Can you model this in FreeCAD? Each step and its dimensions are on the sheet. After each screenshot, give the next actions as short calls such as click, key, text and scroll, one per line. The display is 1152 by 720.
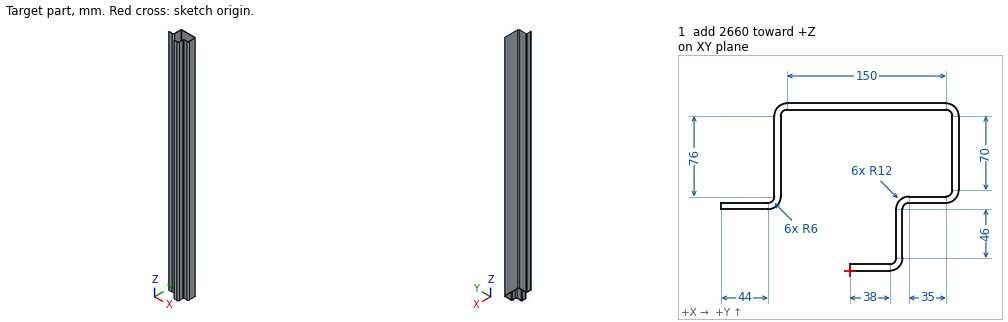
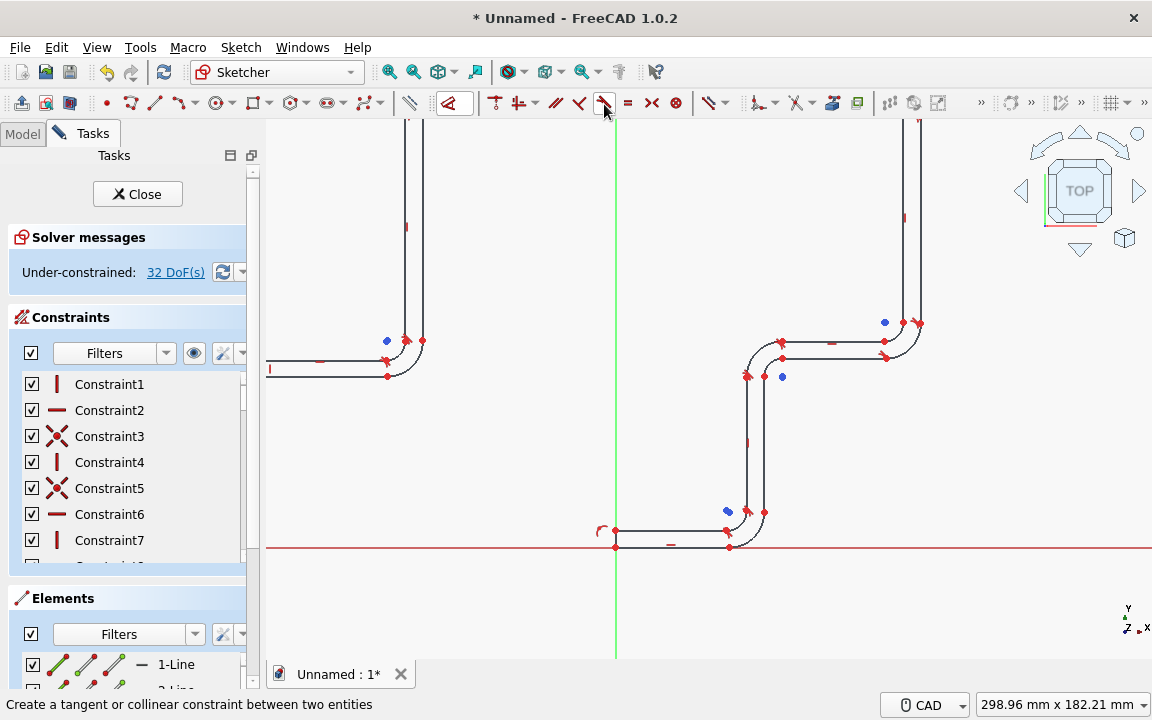
click(813, 359)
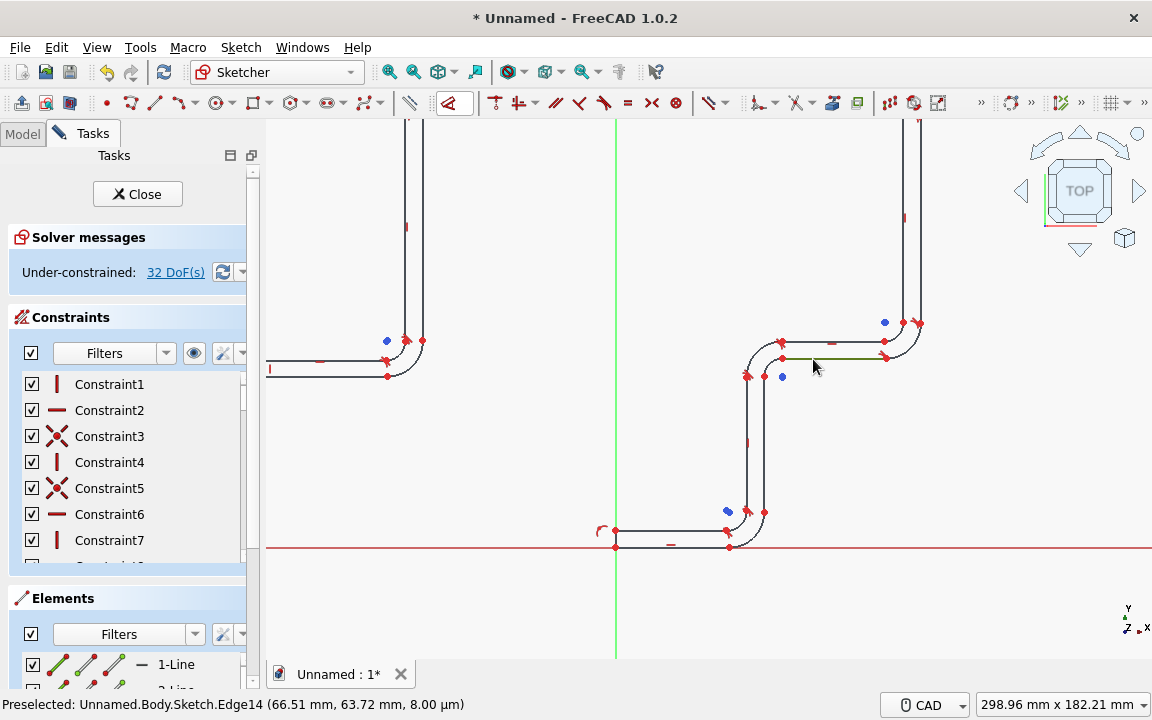
click(902, 355)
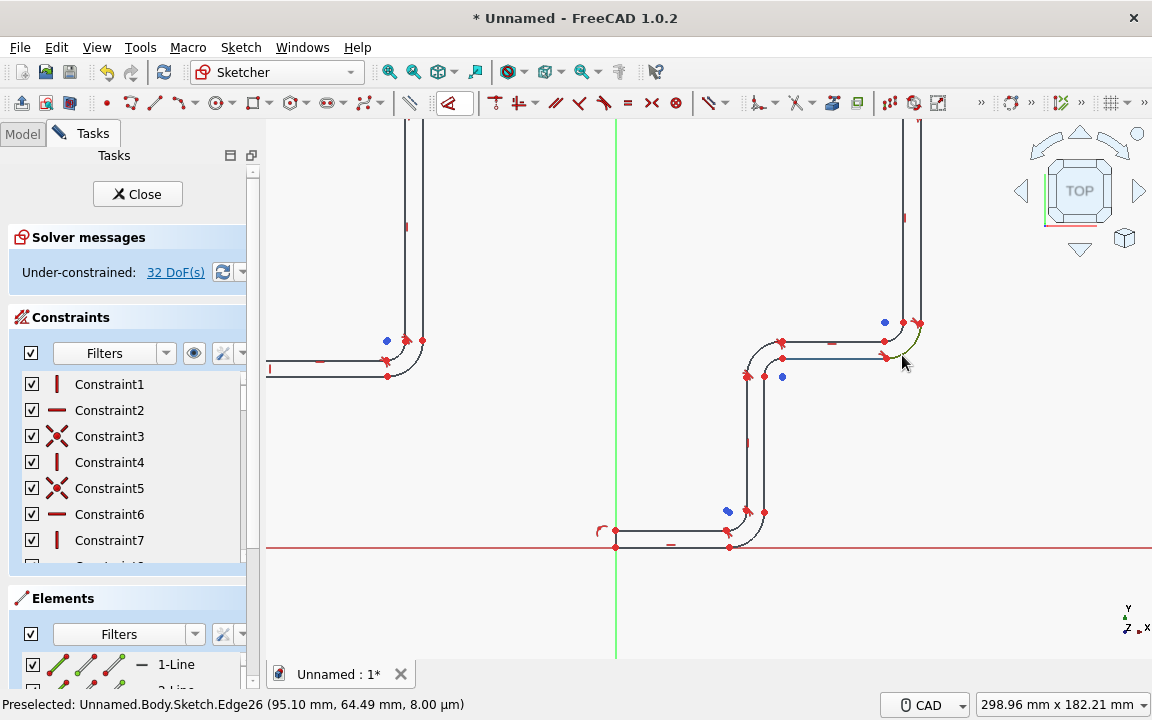
key(t)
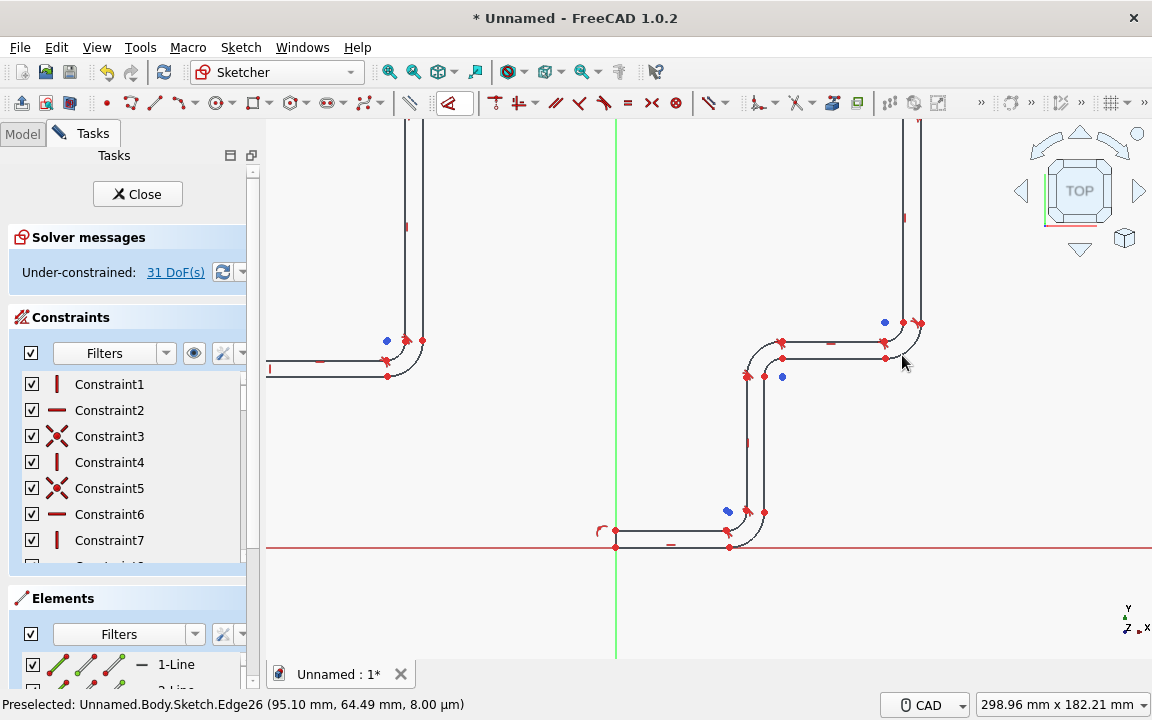
click(921, 261)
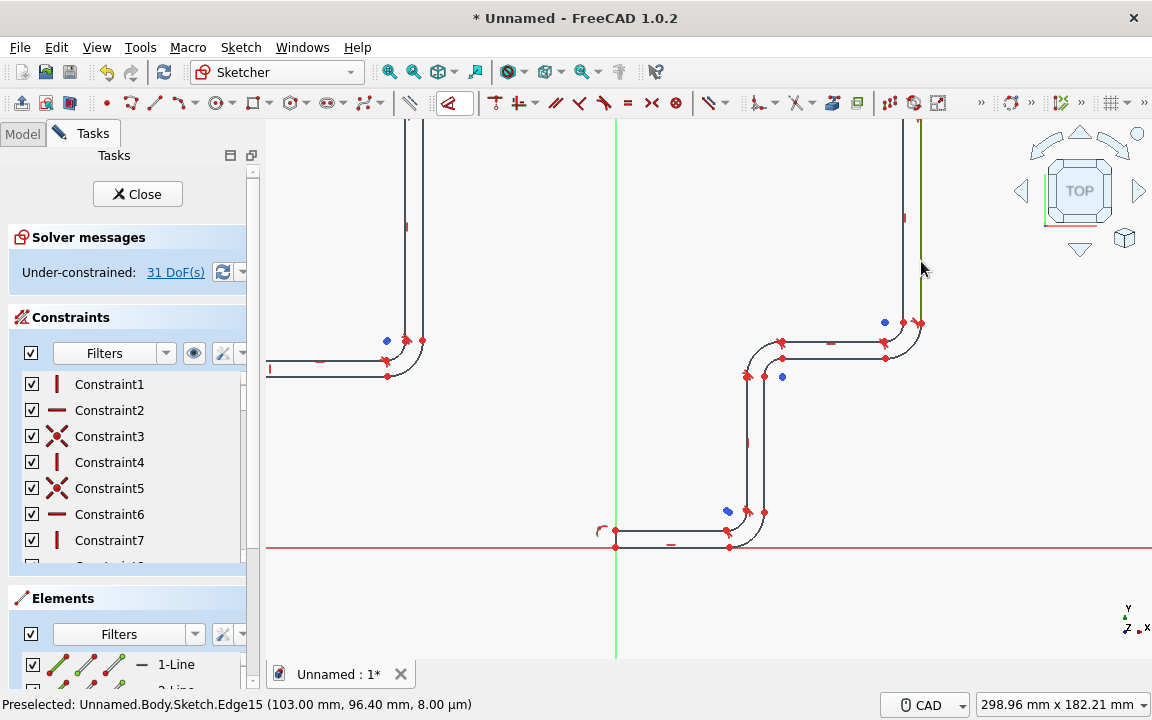
click(901, 355)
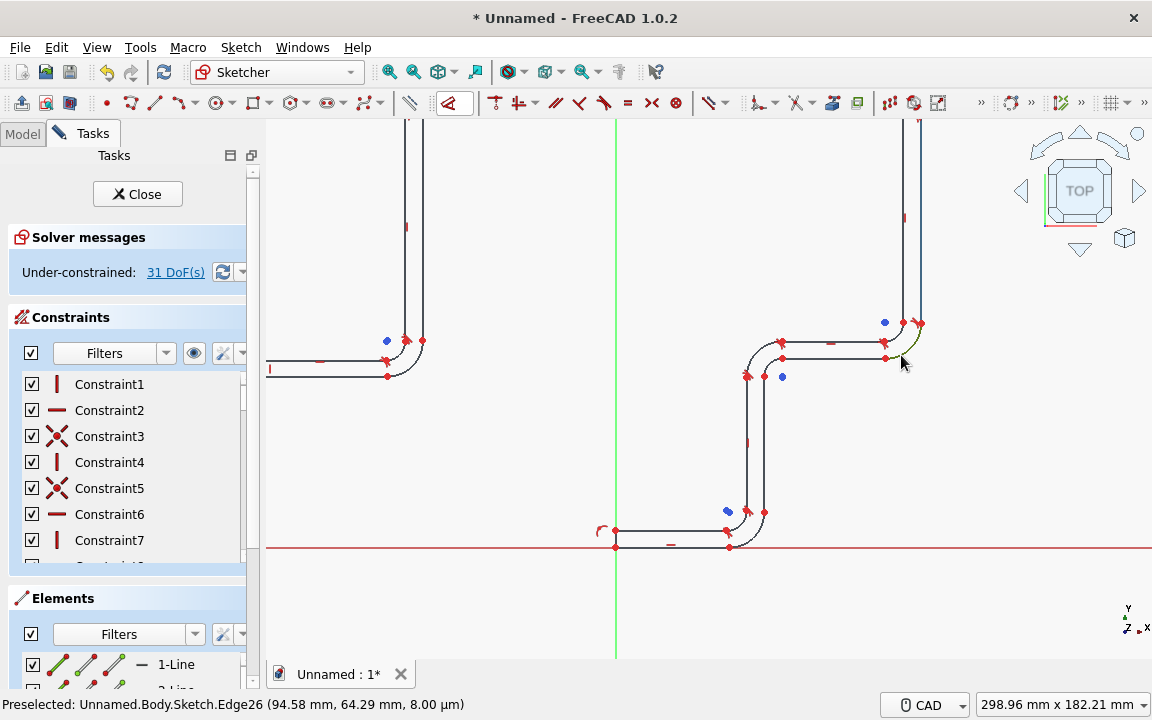
key(t)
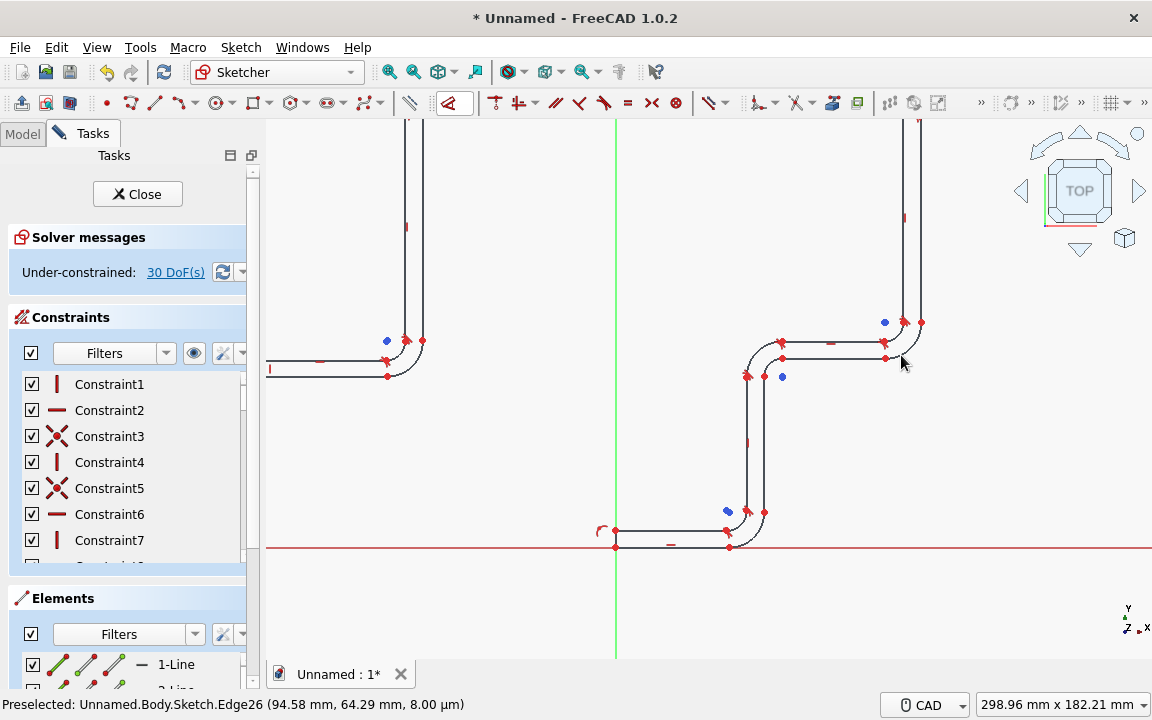
click(921, 261)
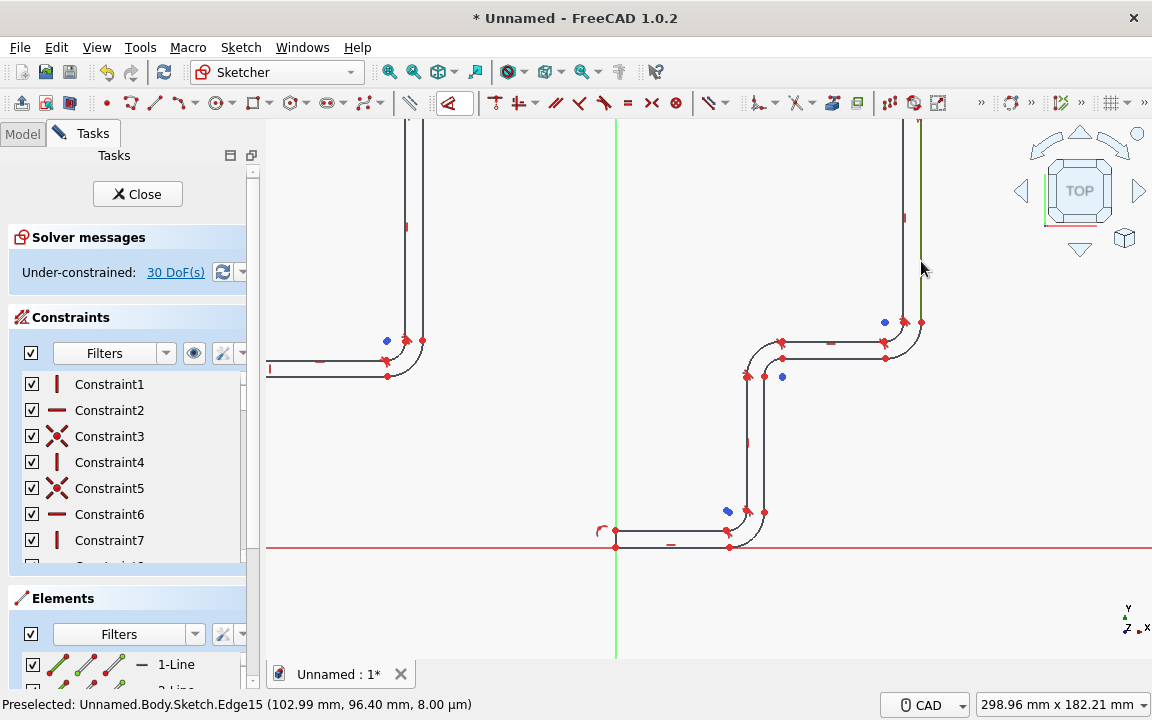
scroll(745, 542, down, 2)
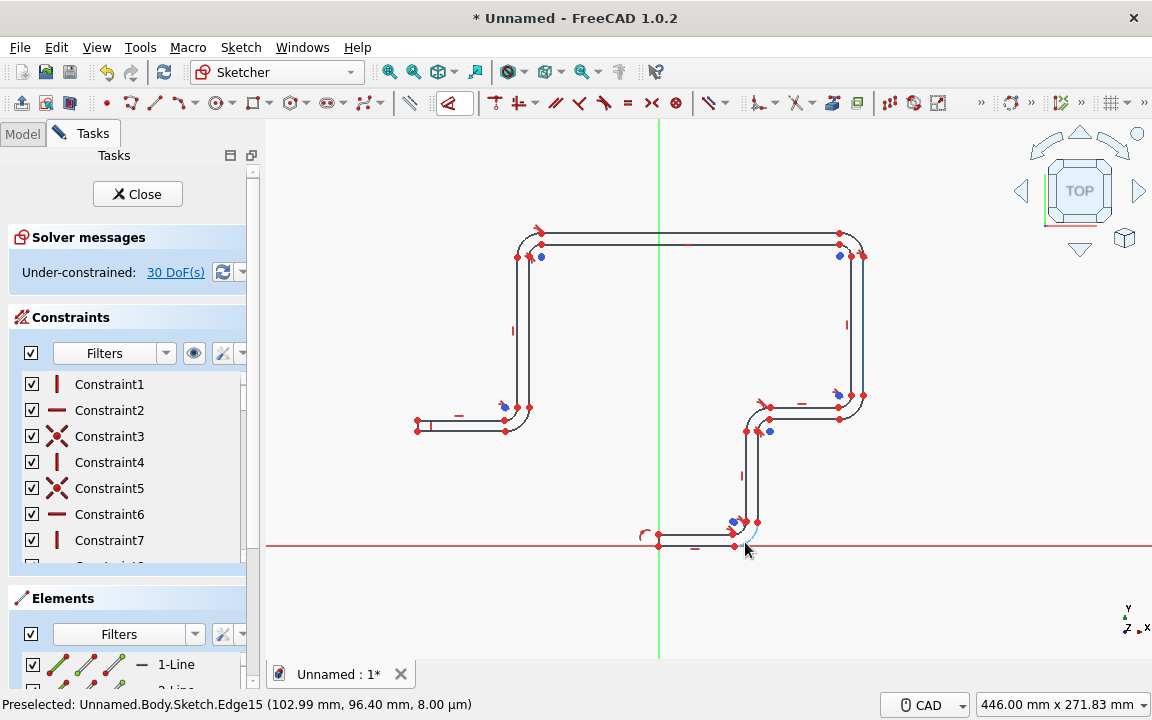
scroll(861, 246, up, 2)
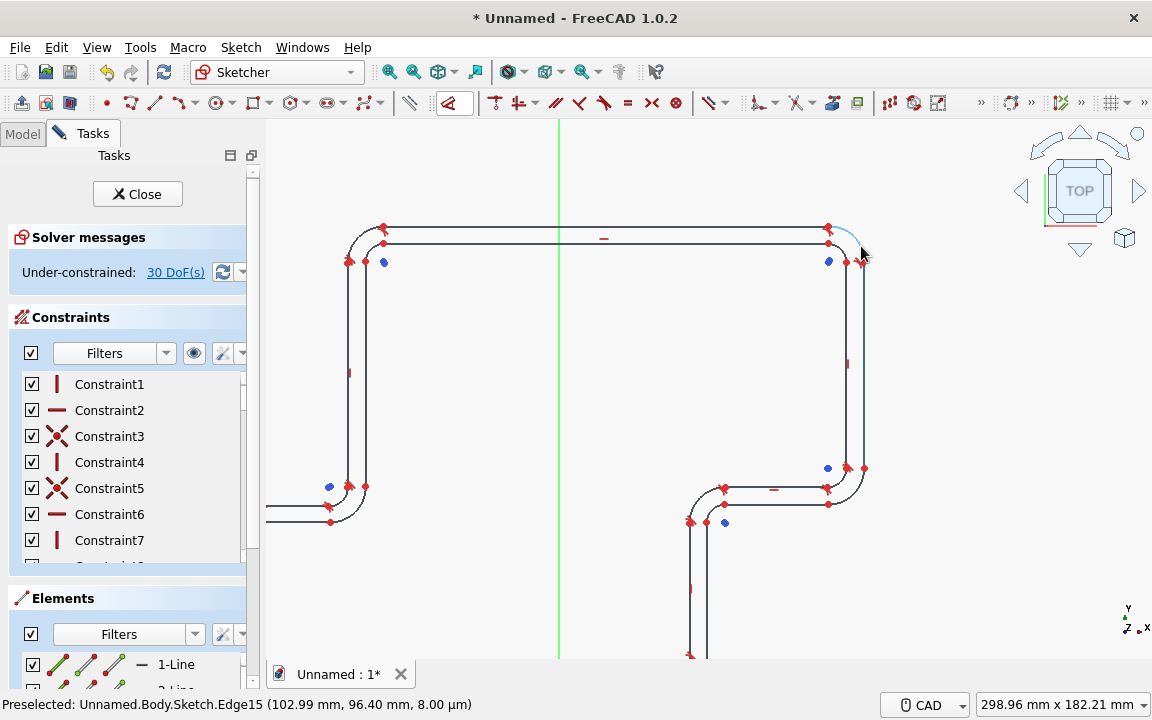
click(861, 246)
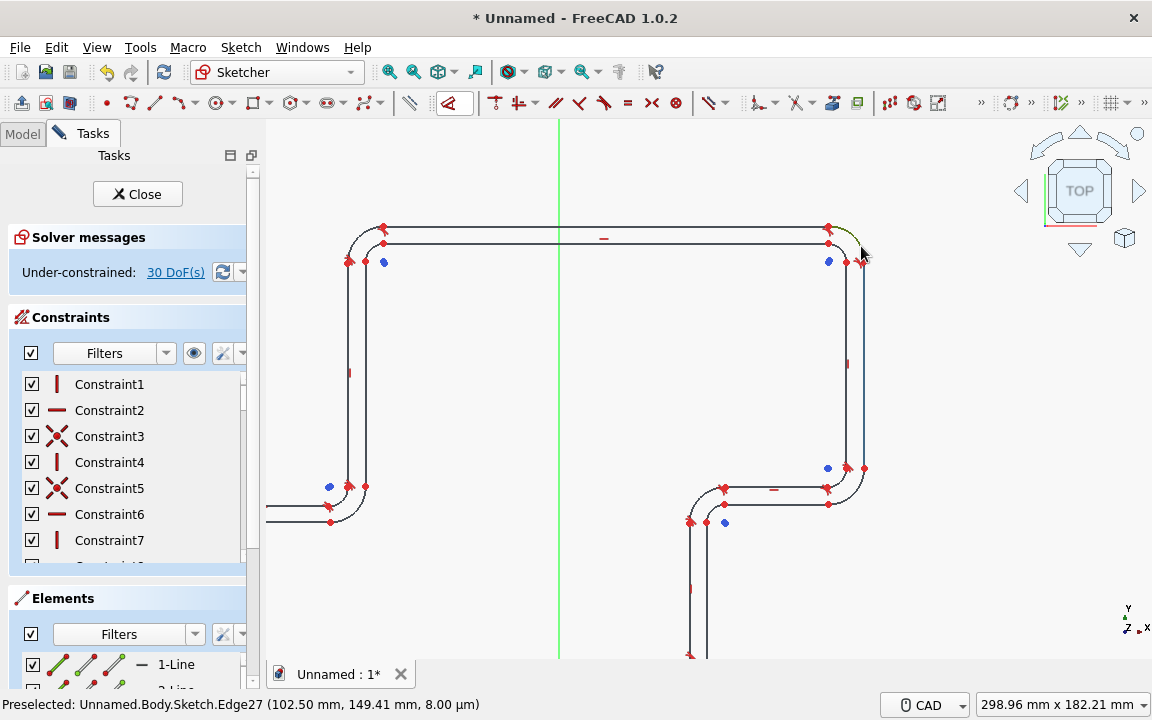
key(t)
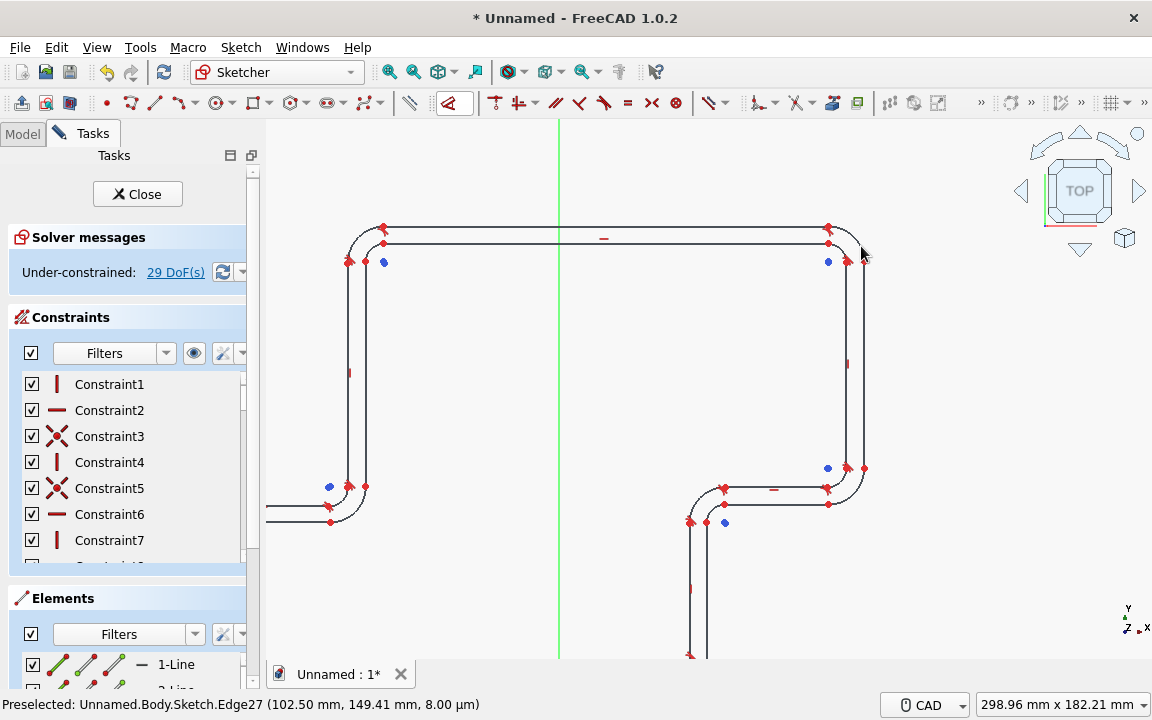
click(695, 227)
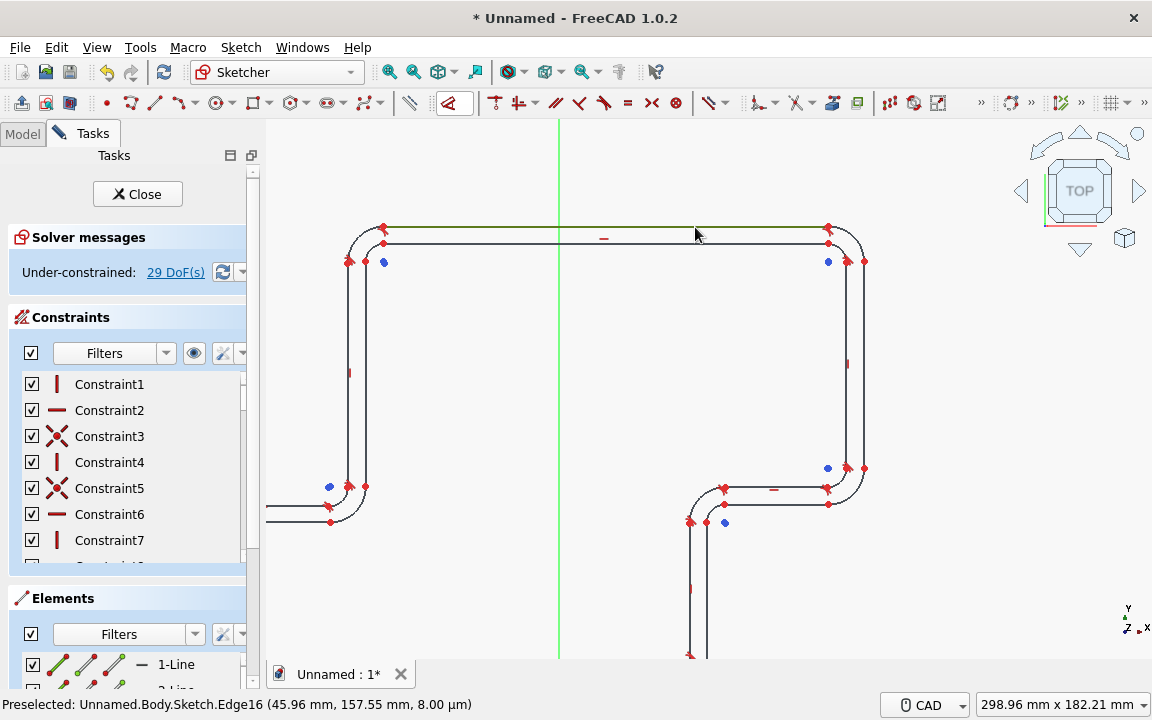
click(860, 246)